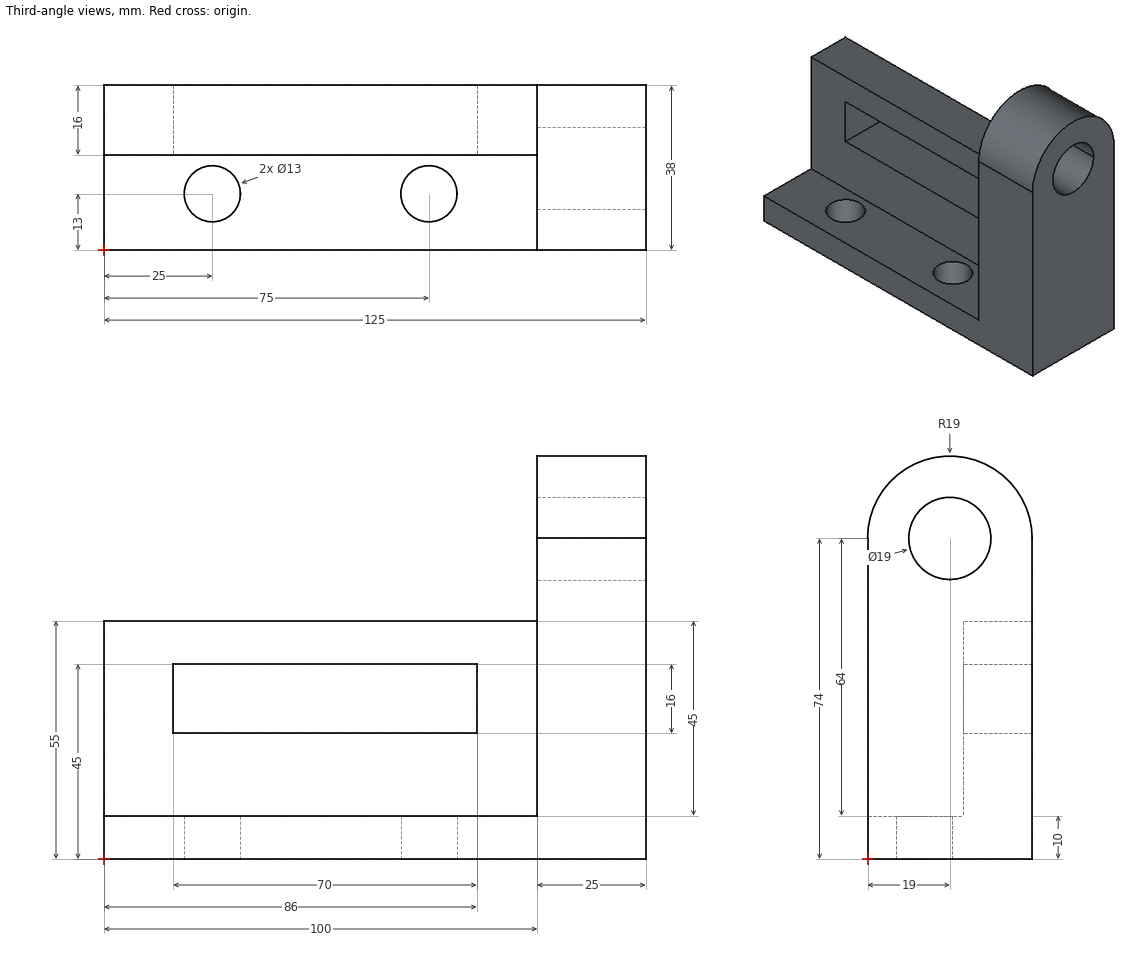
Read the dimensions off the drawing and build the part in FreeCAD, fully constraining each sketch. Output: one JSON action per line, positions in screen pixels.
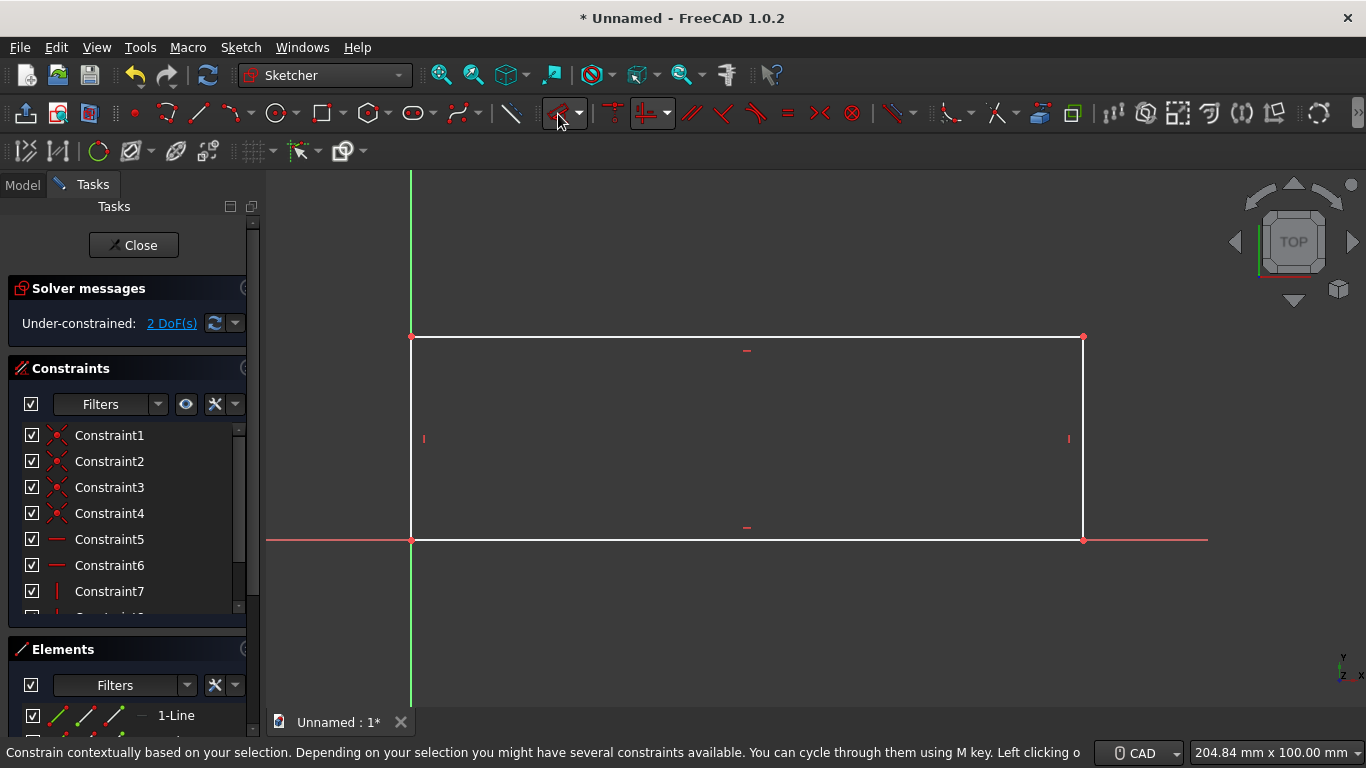
{"action": "left_click", "coordinate": [1083, 479]}
{"action": "left_click", "coordinate": [1117, 439]}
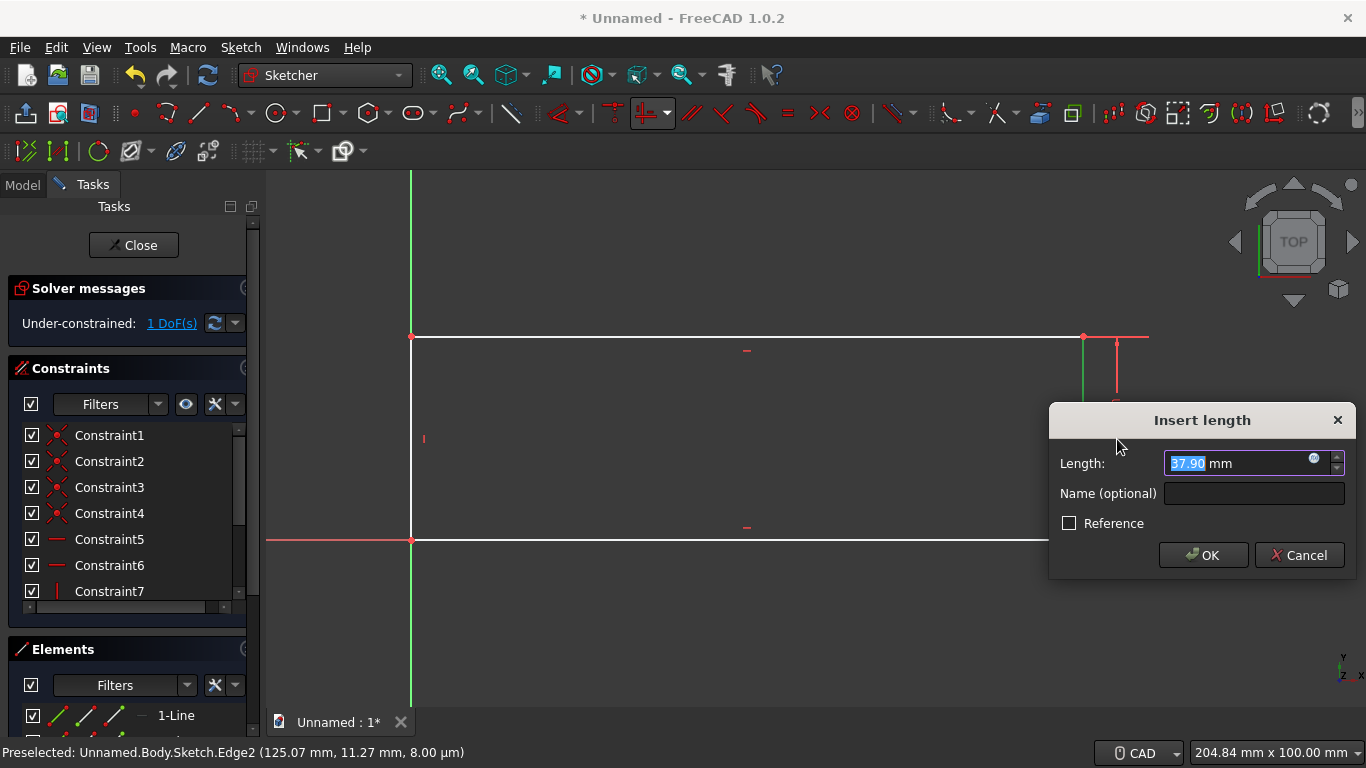
{"action": "type", "text": "38"}
{"action": "key", "text": "Return"}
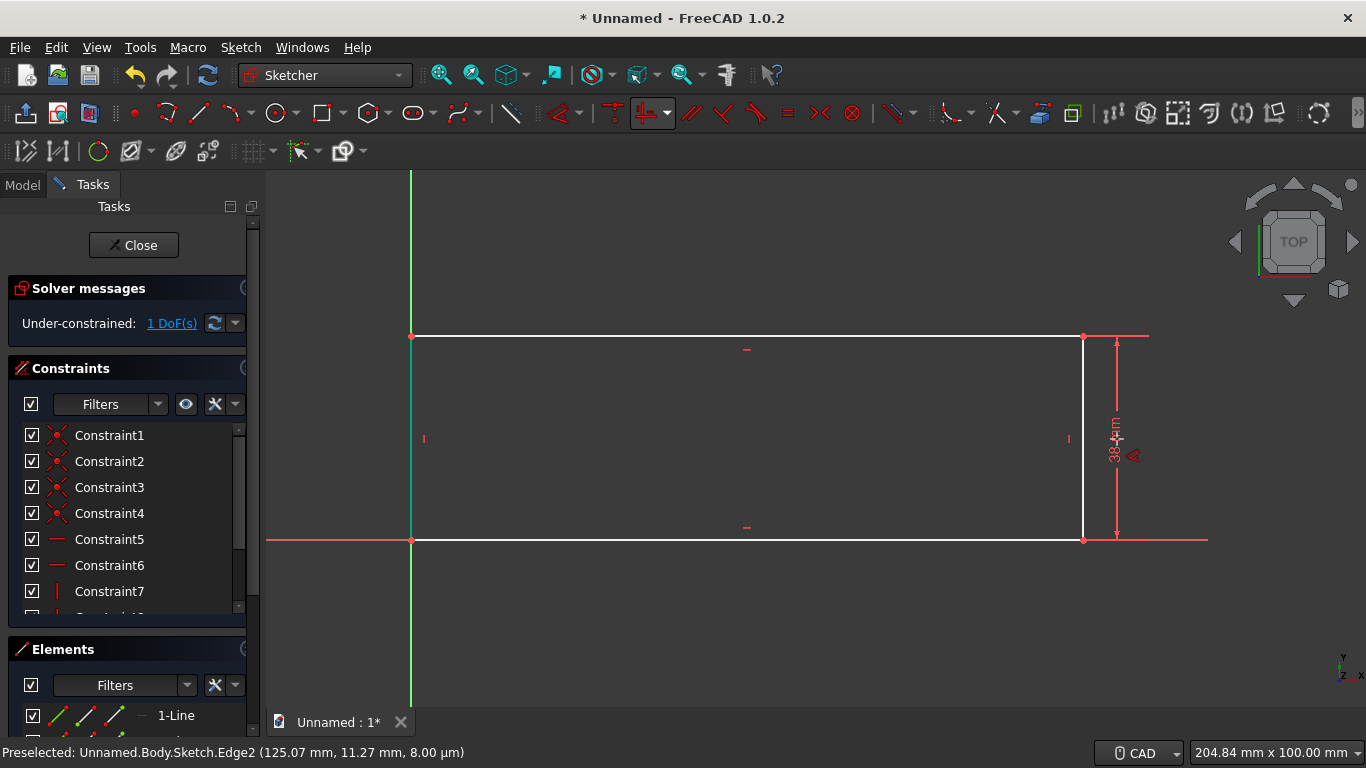
{"action": "left_click", "coordinate": [613, 540]}
{"action": "left_click", "coordinate": [747, 574]}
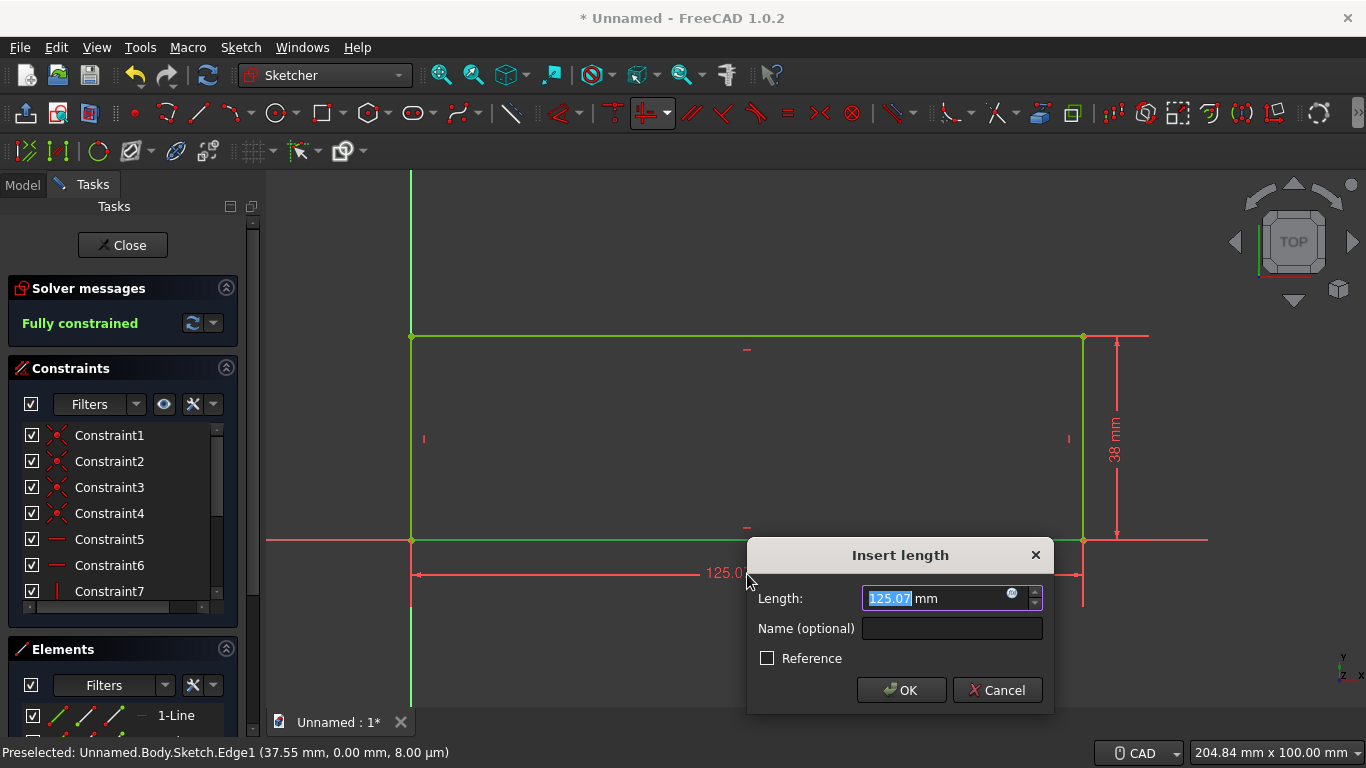
{"action": "type", "text": "125"}
{"action": "key", "text": "Return"}
{"action": "key", "text": "Escape"}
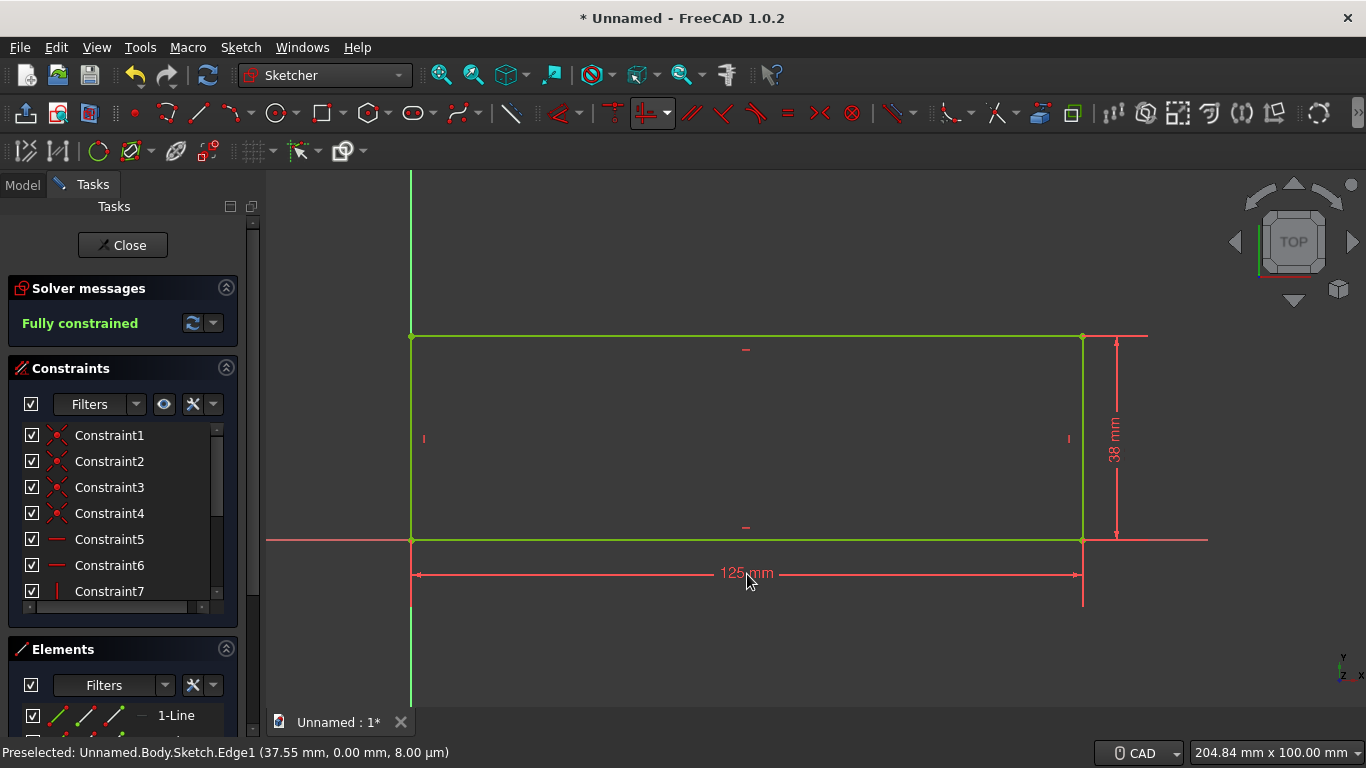
{"action": "left_click", "coordinate": [123, 245]}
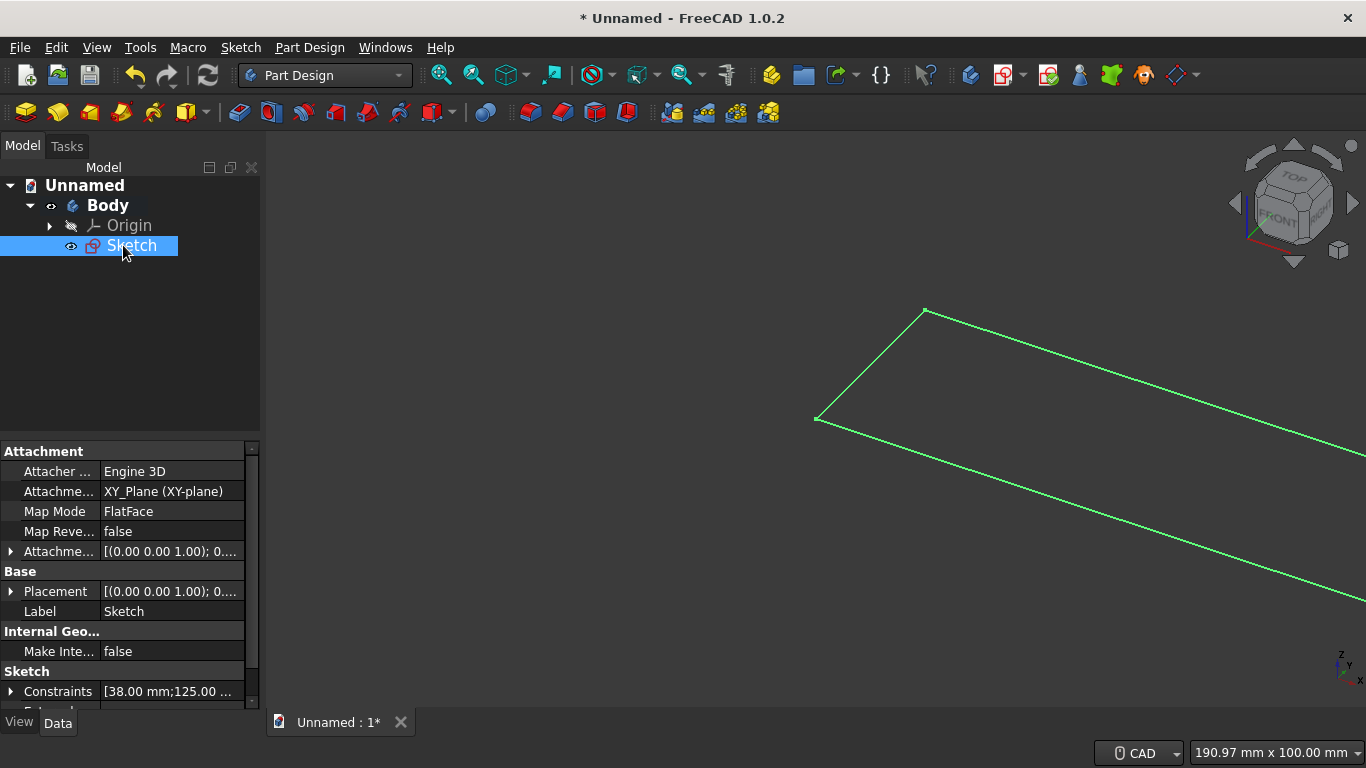
{"action": "left_click", "coordinate": [26, 112]}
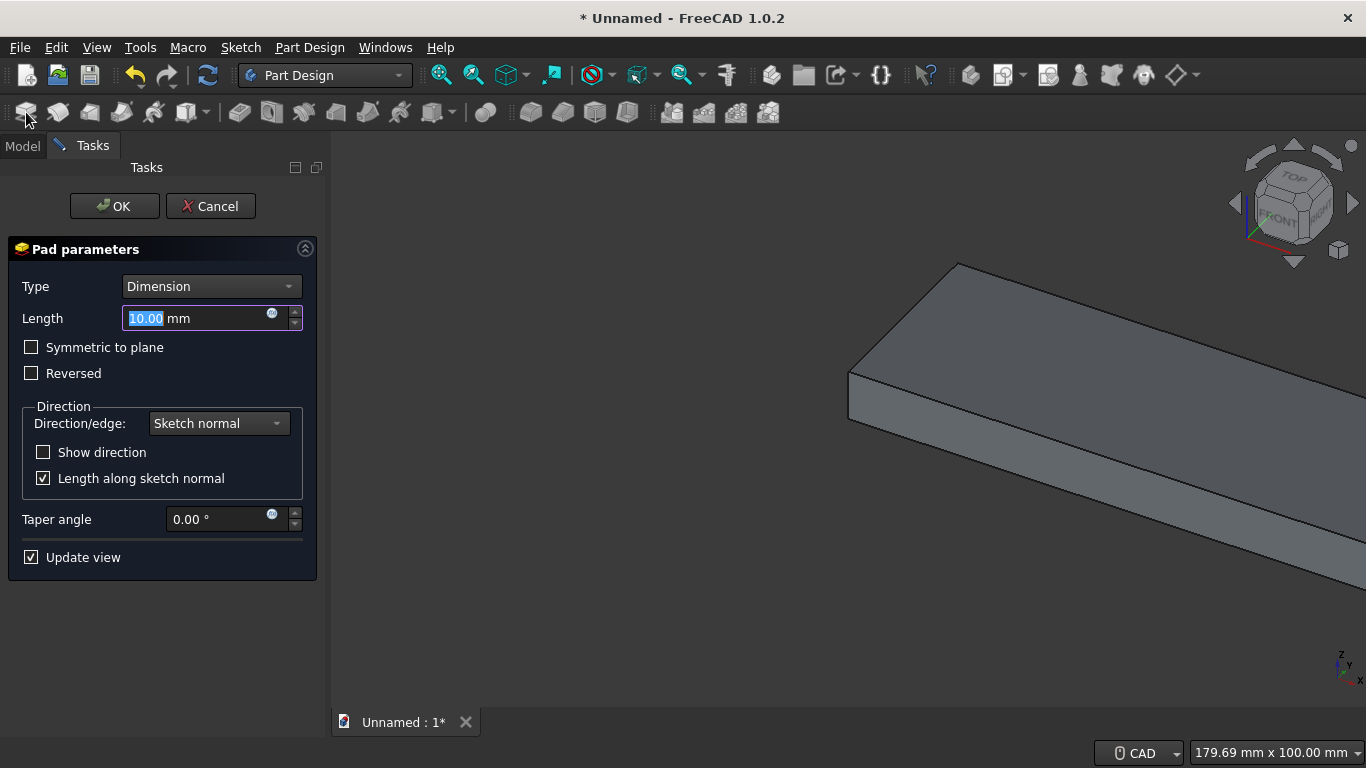
{"action": "type", "text": "10"}
{"action": "key", "text": "Tab"}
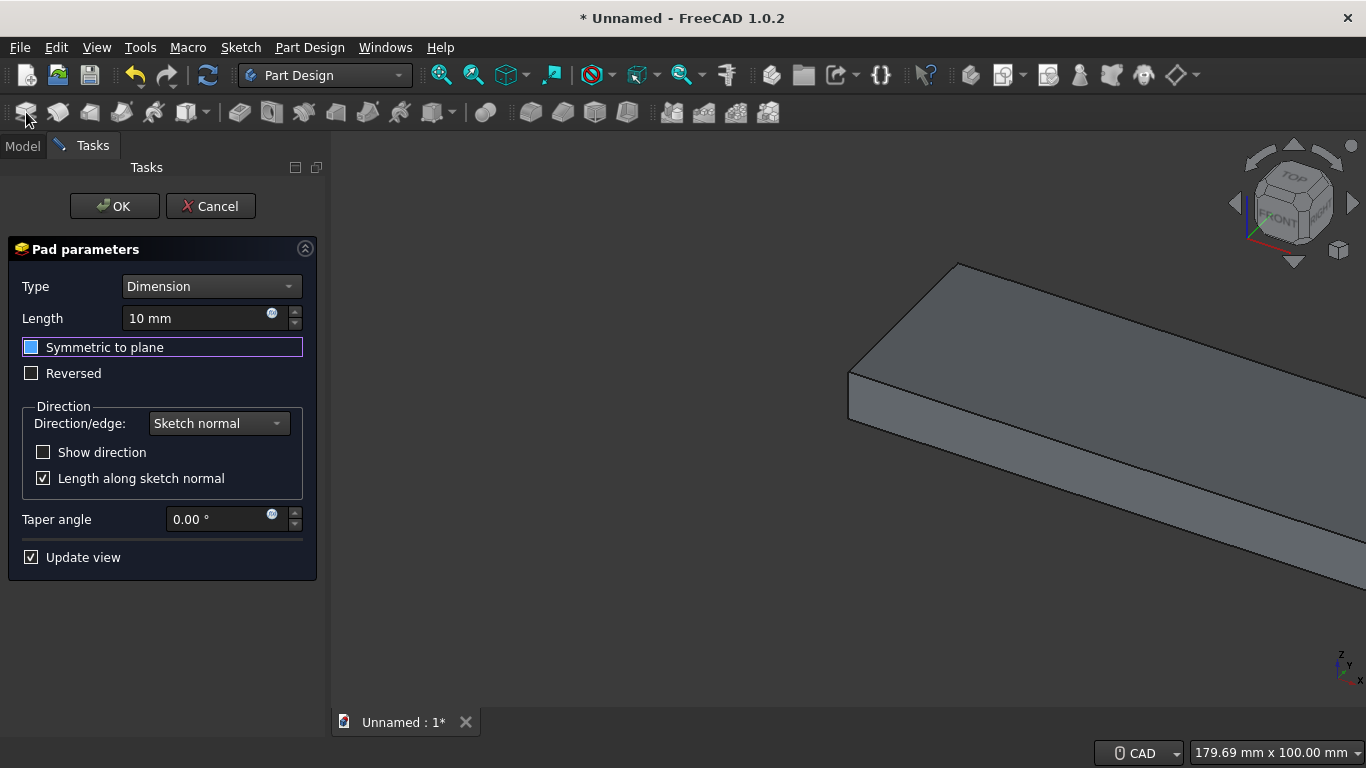
{"action": "left_click", "coordinate": [115, 206]}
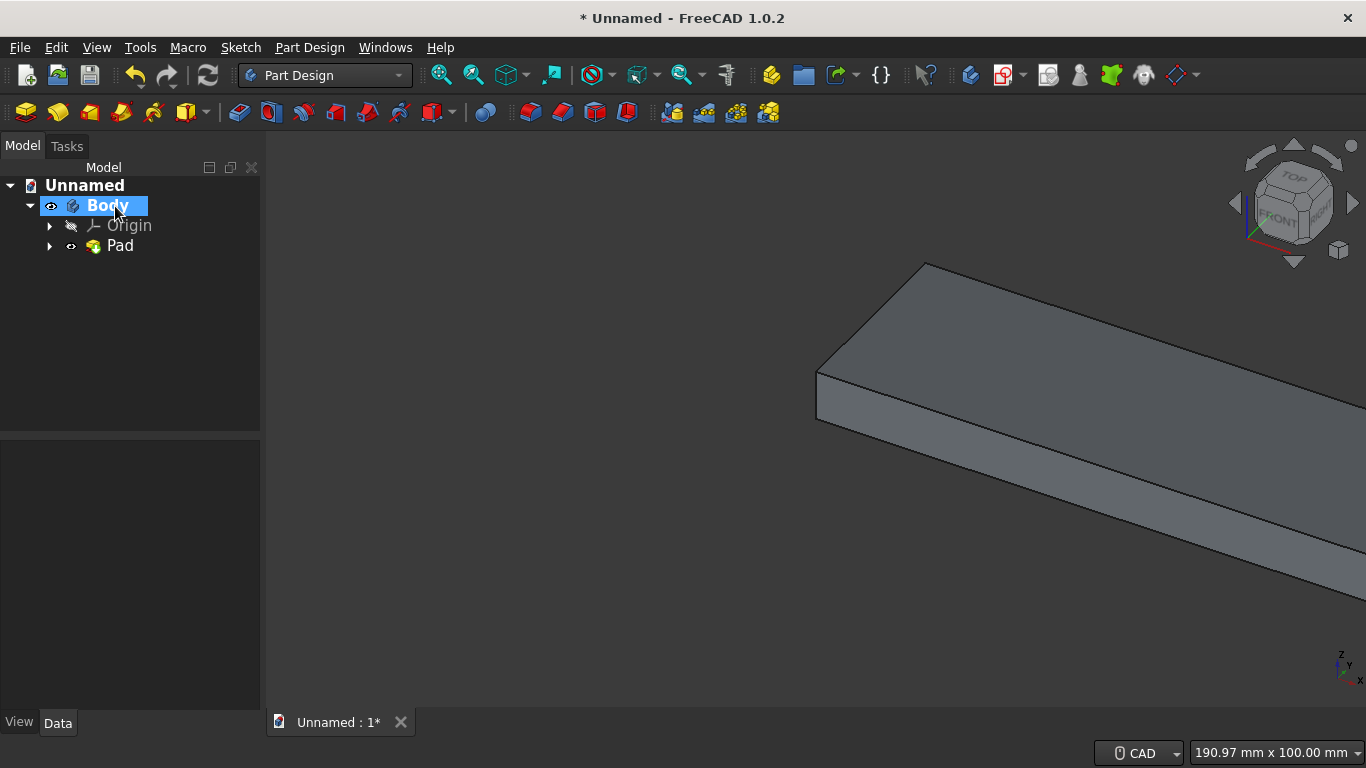
{"action": "left_click", "coordinate": [442, 76]}